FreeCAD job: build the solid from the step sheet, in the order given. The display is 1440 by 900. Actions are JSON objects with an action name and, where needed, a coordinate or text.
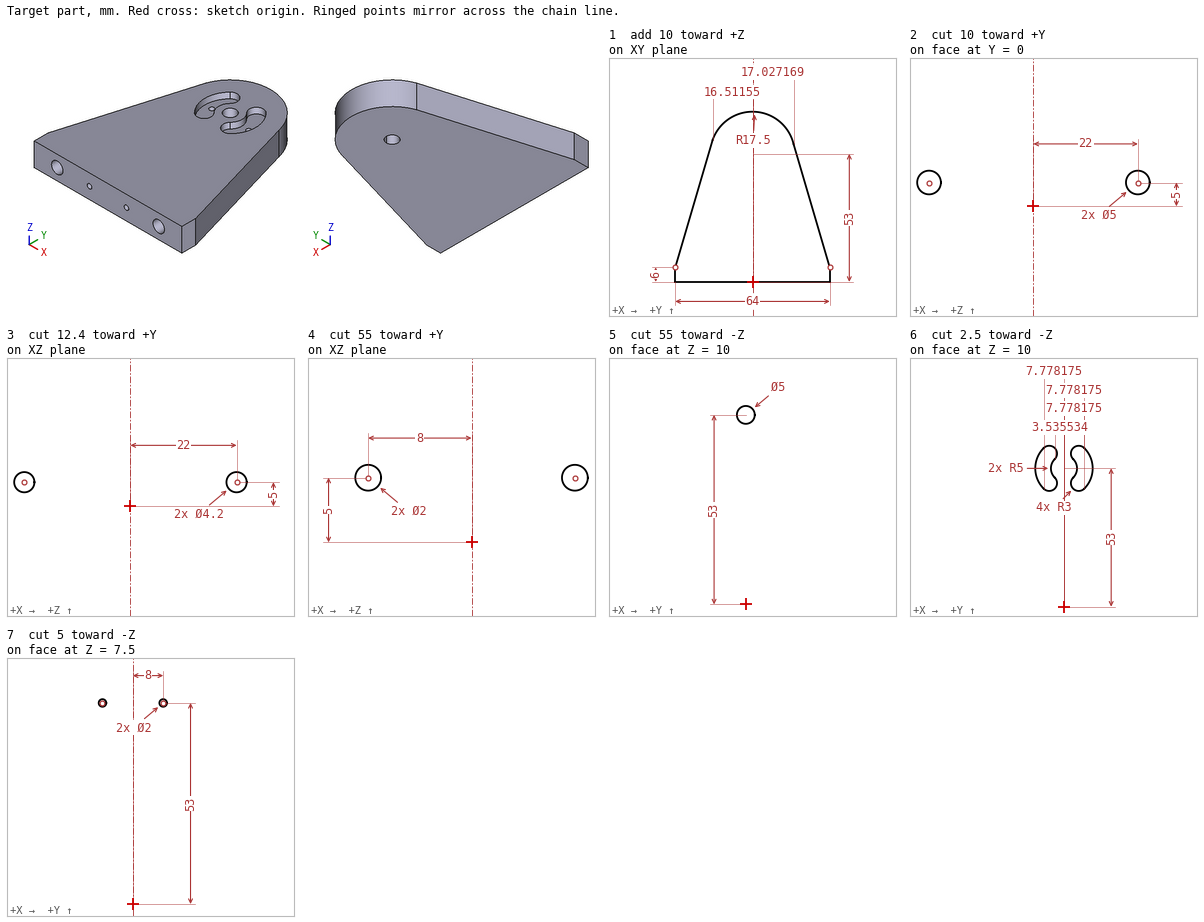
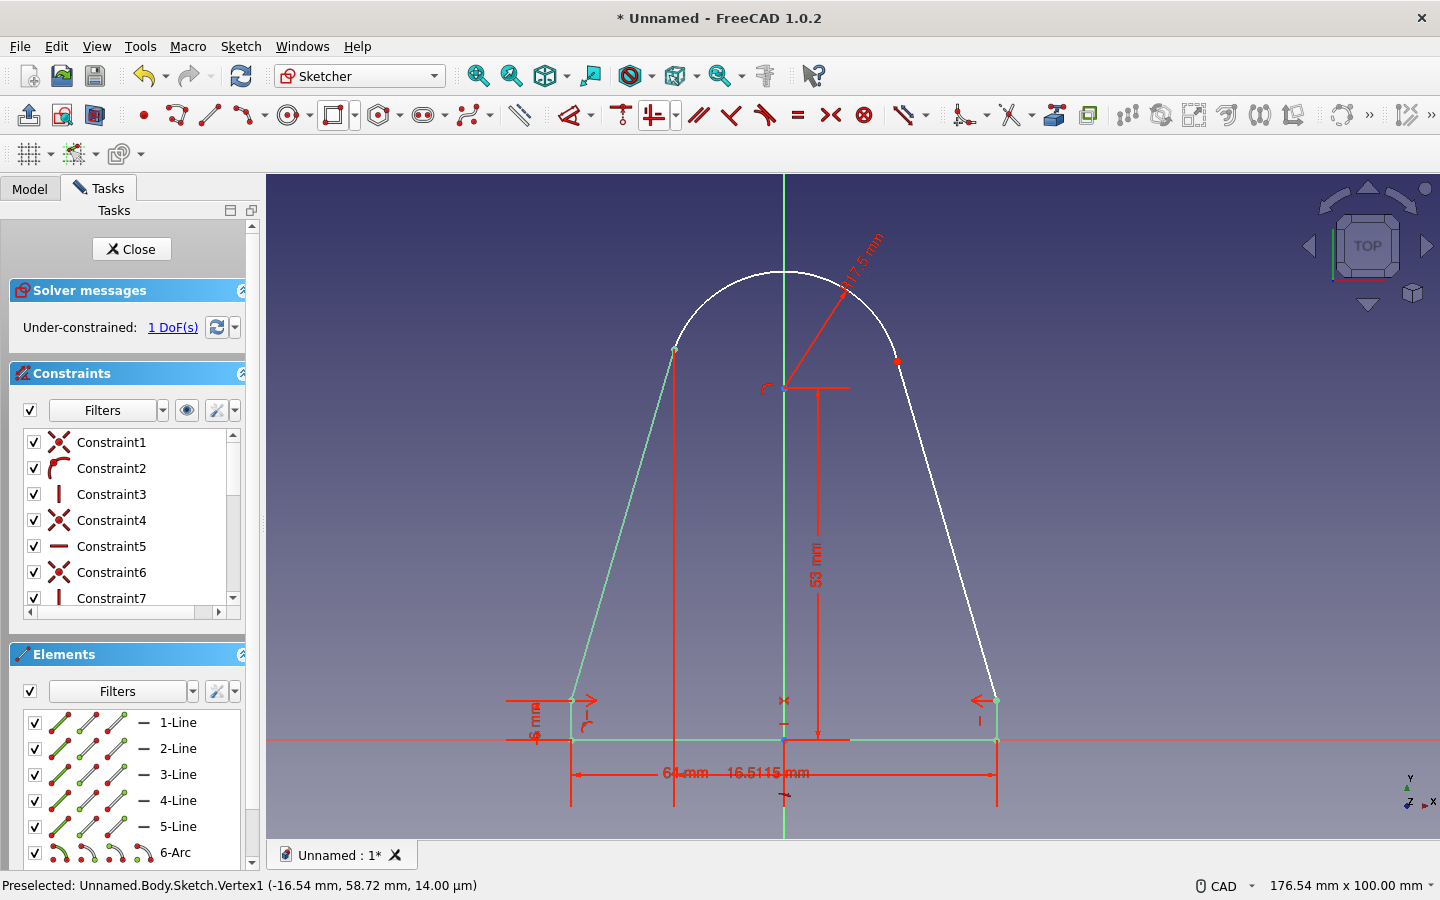
{"action": "left_click", "coordinate": [898, 362]}
{"action": "left_click", "coordinate": [841, 774]}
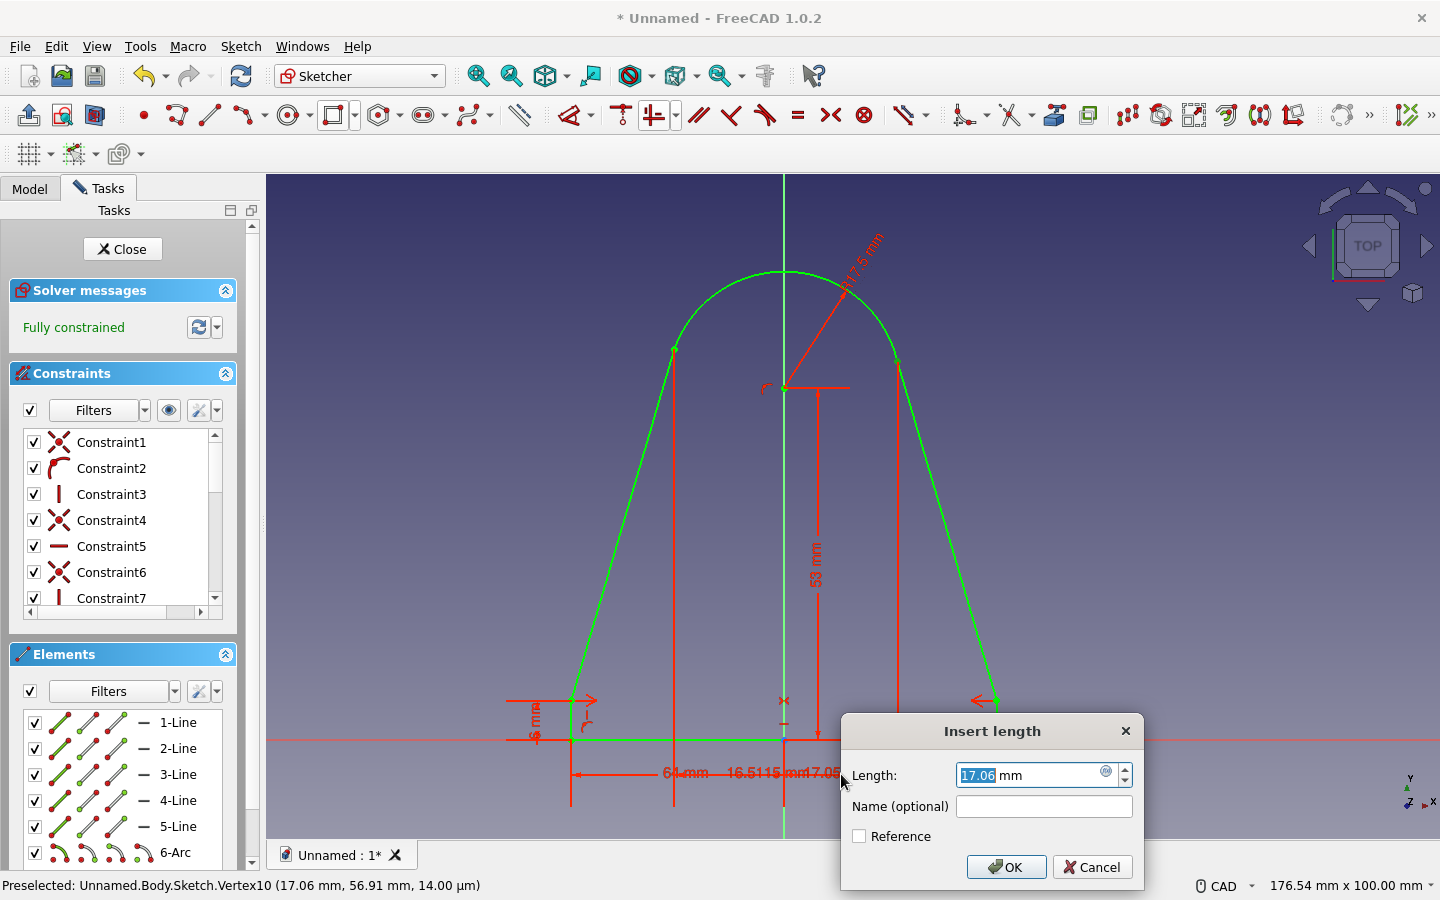
{"action": "type", "text": "17.027169"}
{"action": "key", "text": "Return"}
{"action": "key", "text": "Escape"}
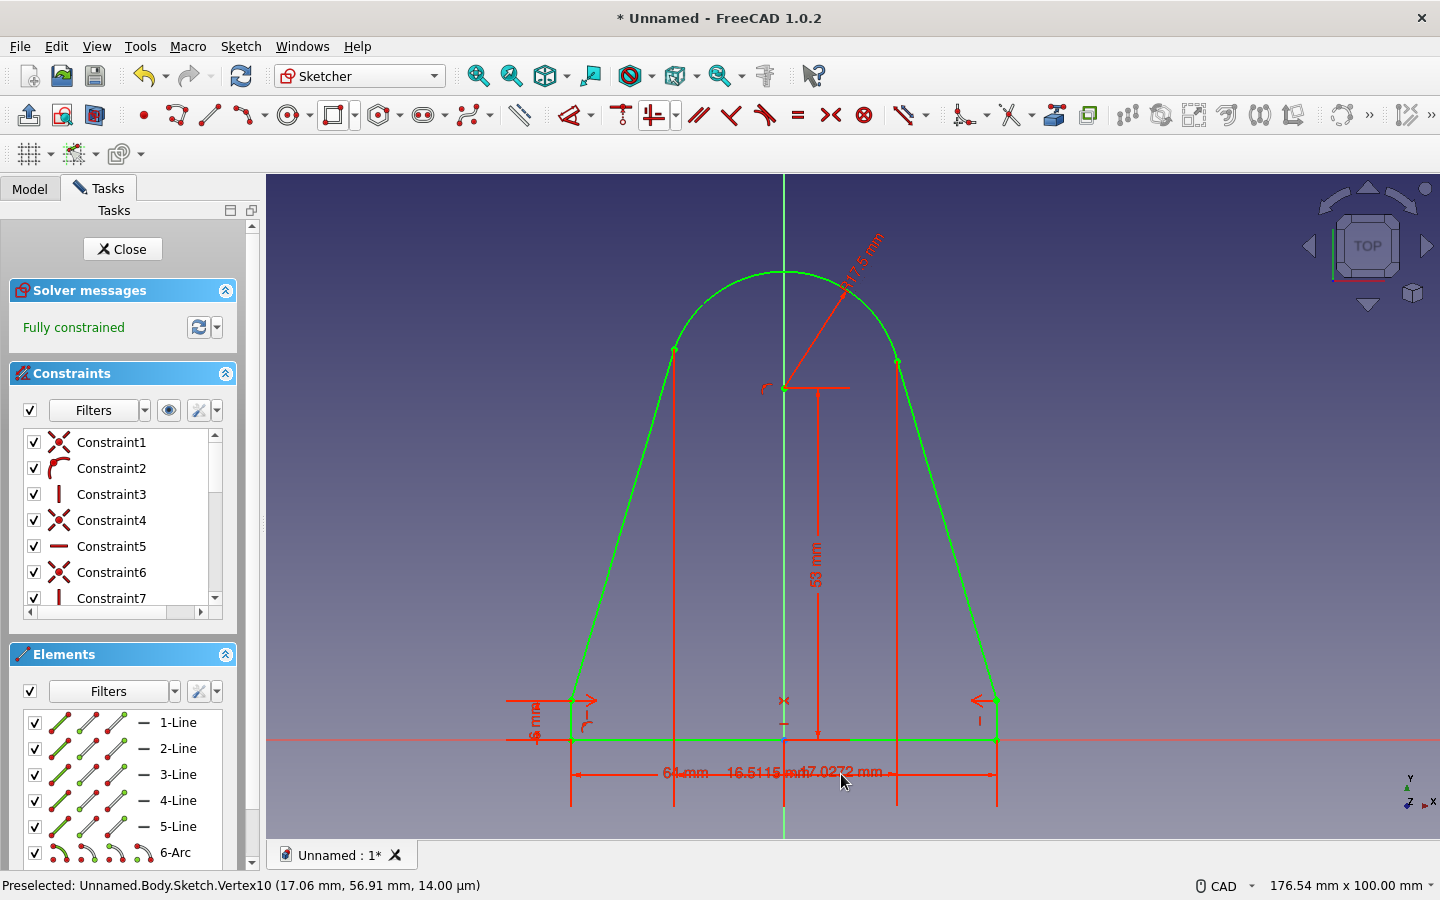
{"action": "left_click", "coordinate": [123, 249]}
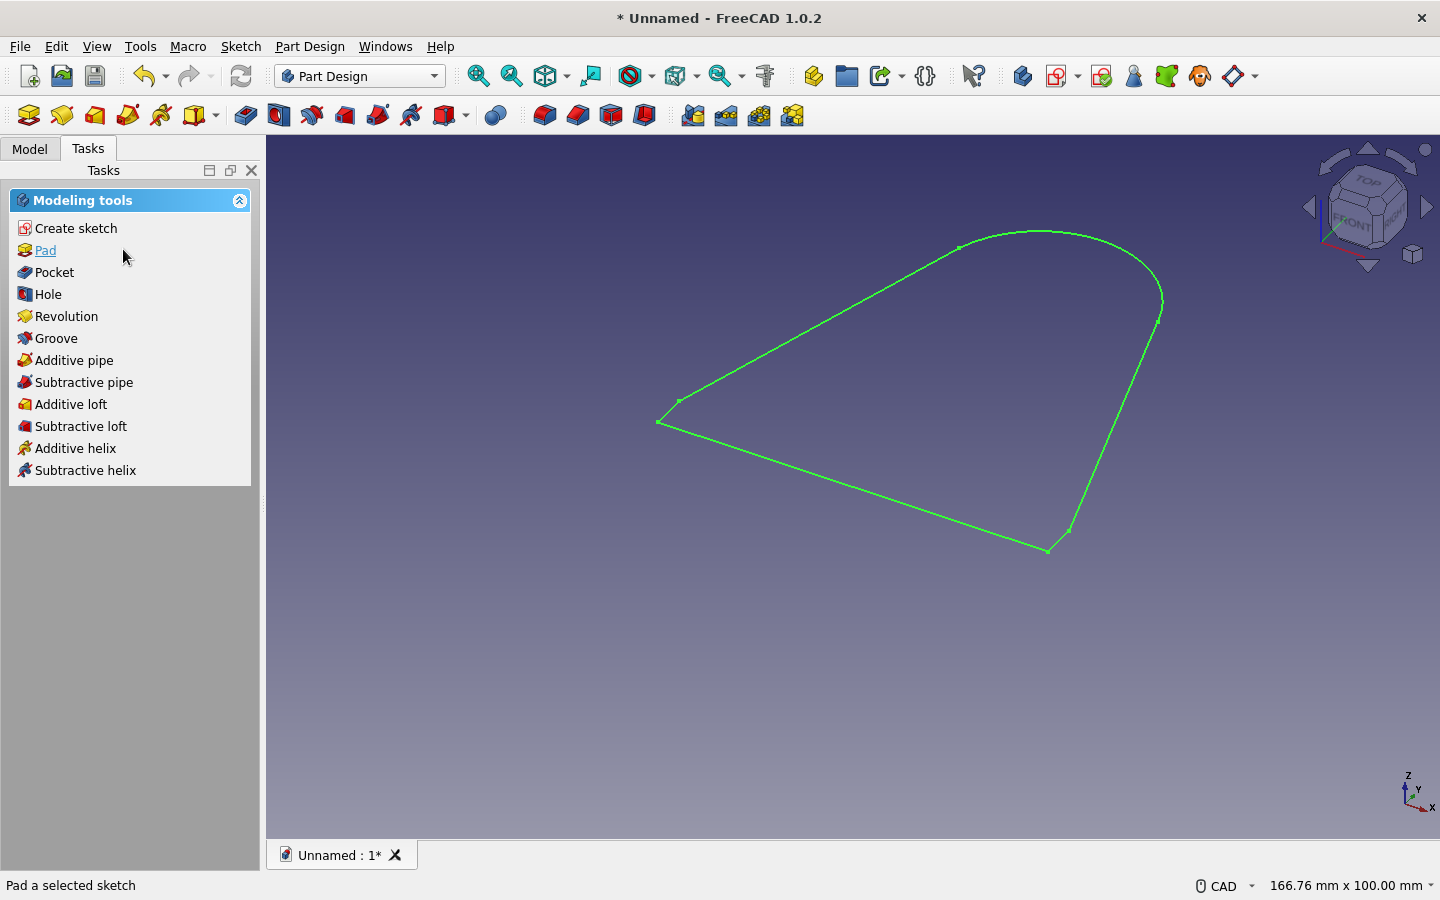
{"action": "left_click", "coordinate": [29, 116]}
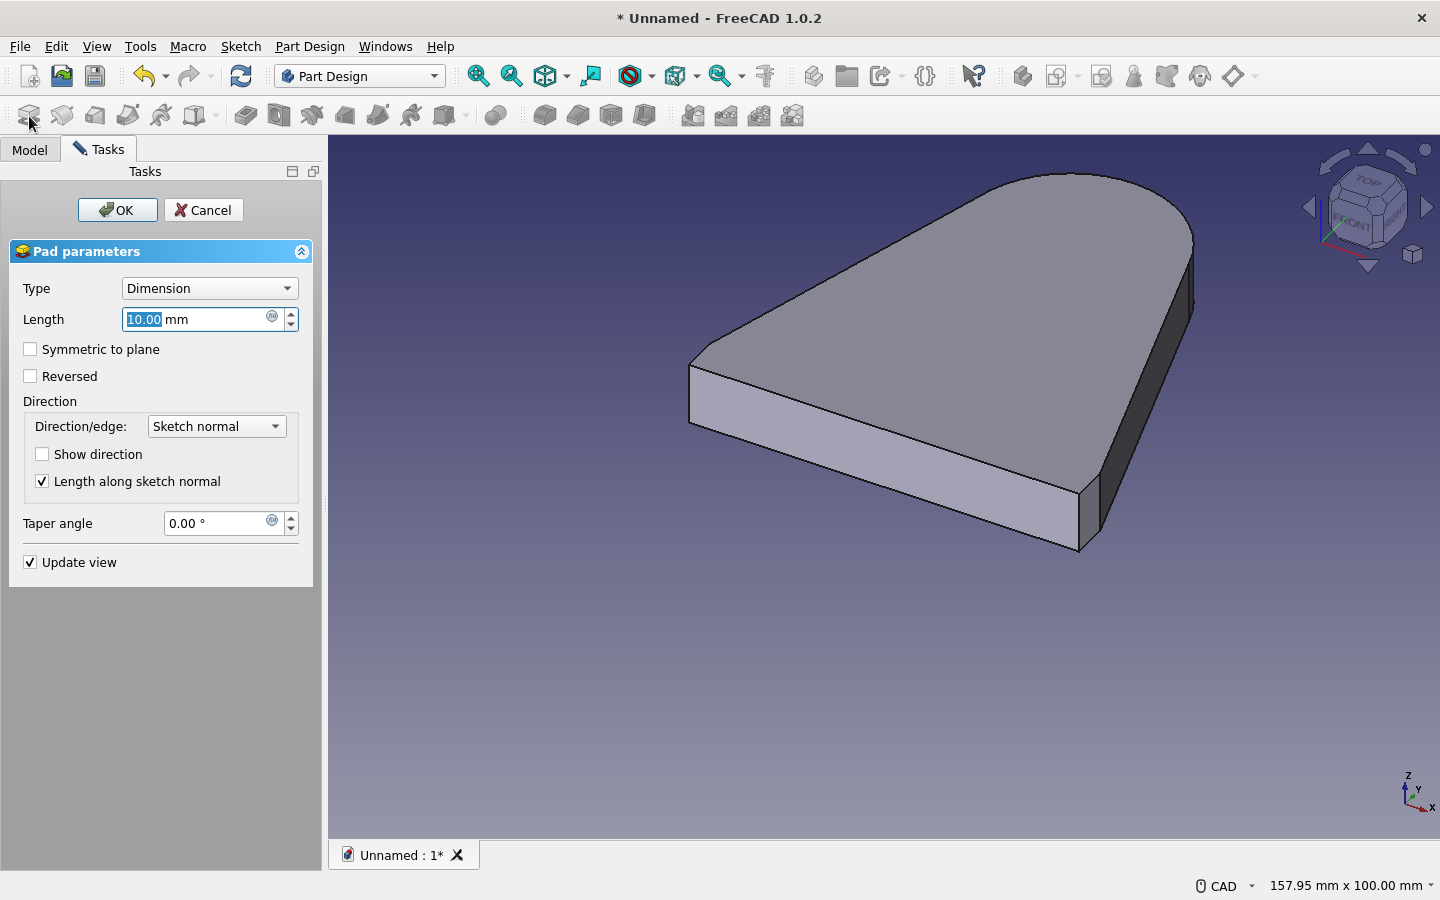
{"action": "type", "text": "10"}
{"action": "key", "text": "Tab"}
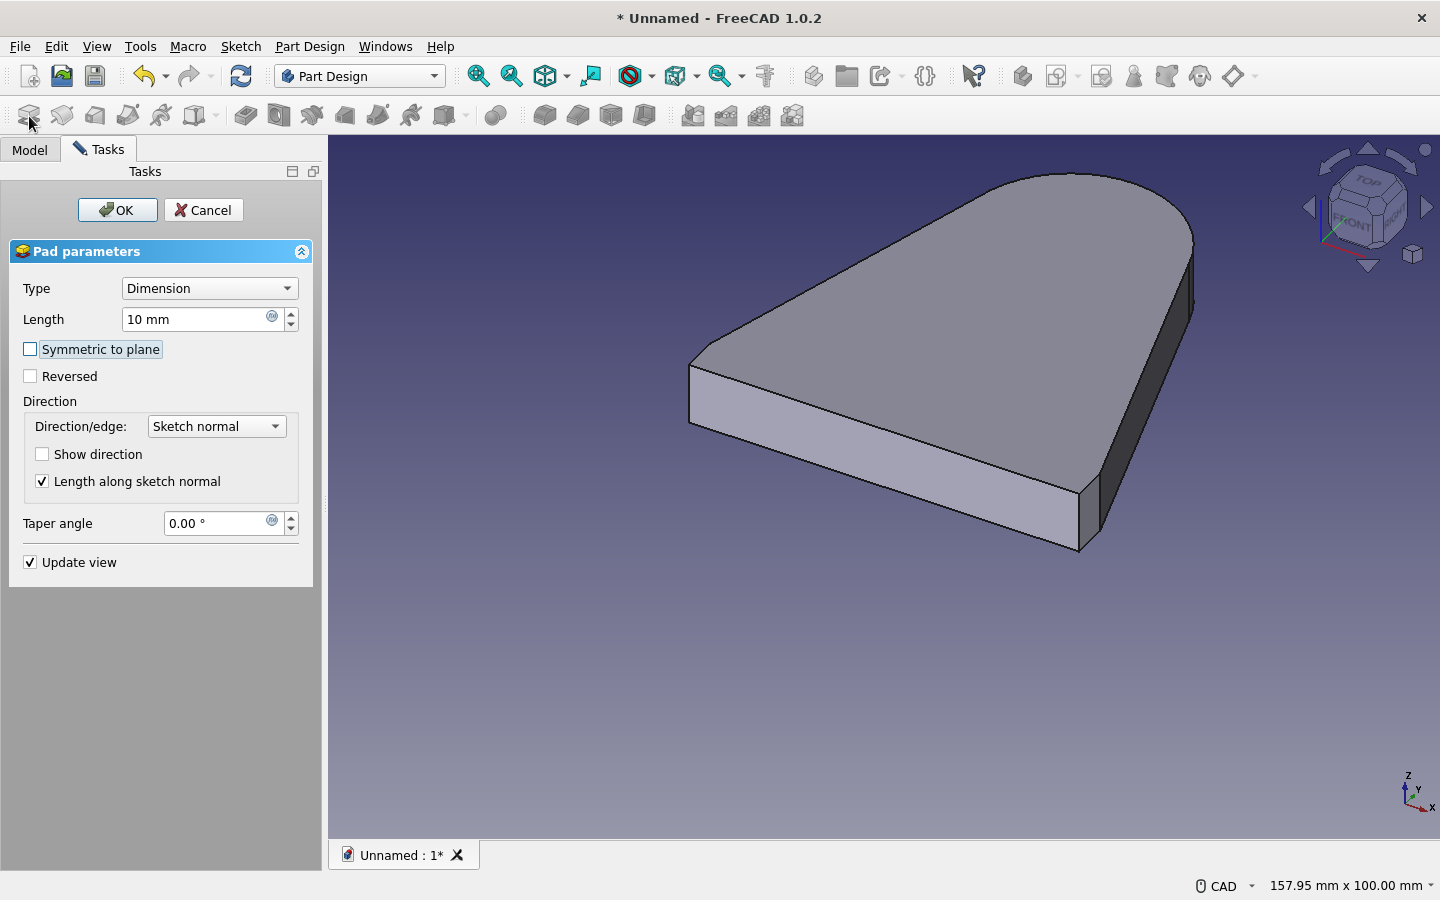
{"action": "left_click", "coordinate": [118, 210]}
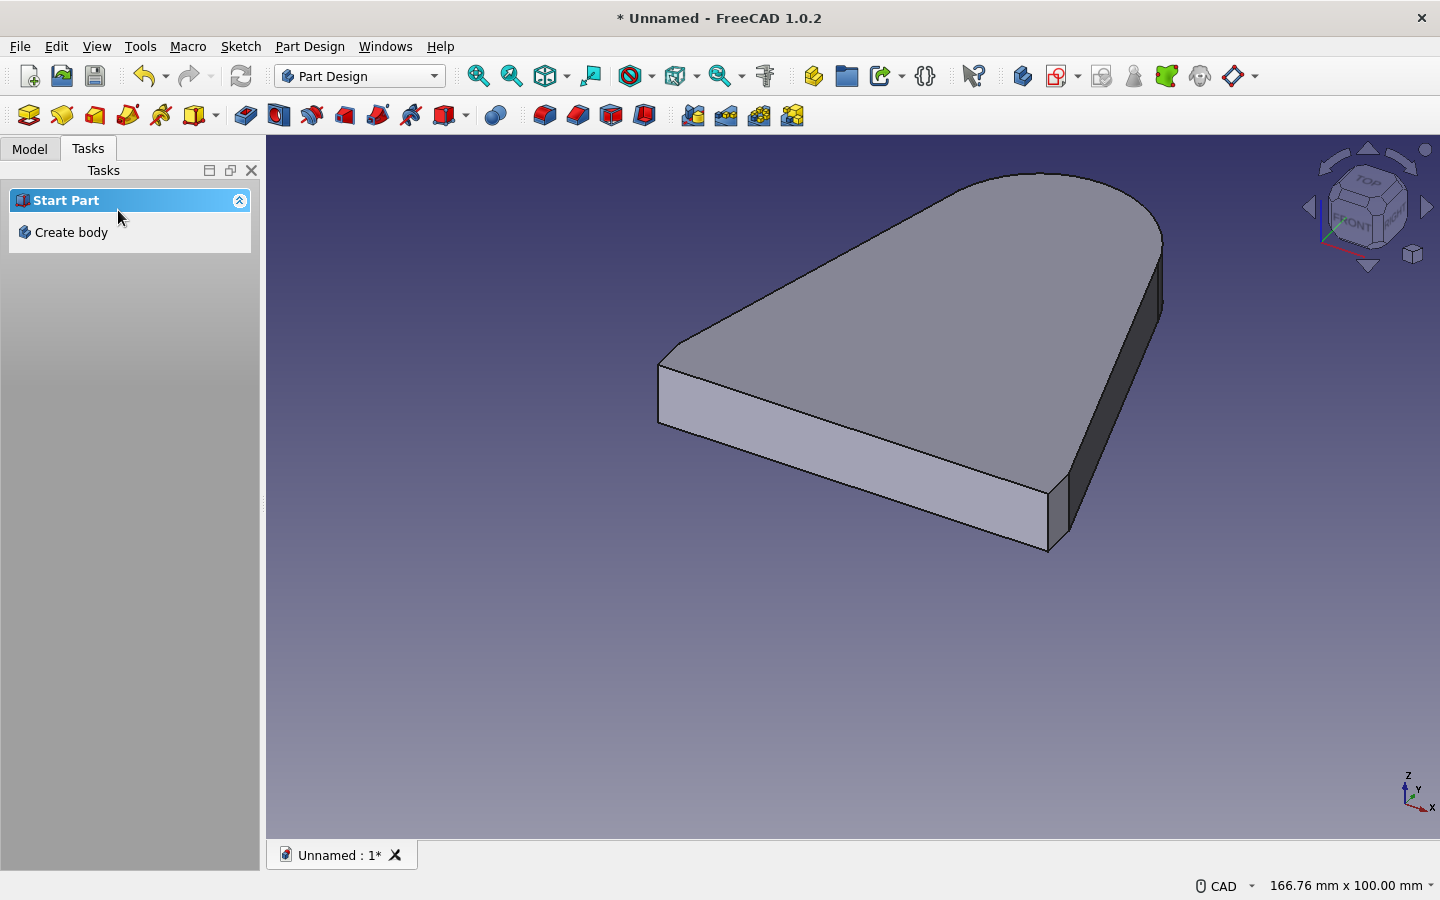
{"action": "left_click", "coordinate": [479, 76]}